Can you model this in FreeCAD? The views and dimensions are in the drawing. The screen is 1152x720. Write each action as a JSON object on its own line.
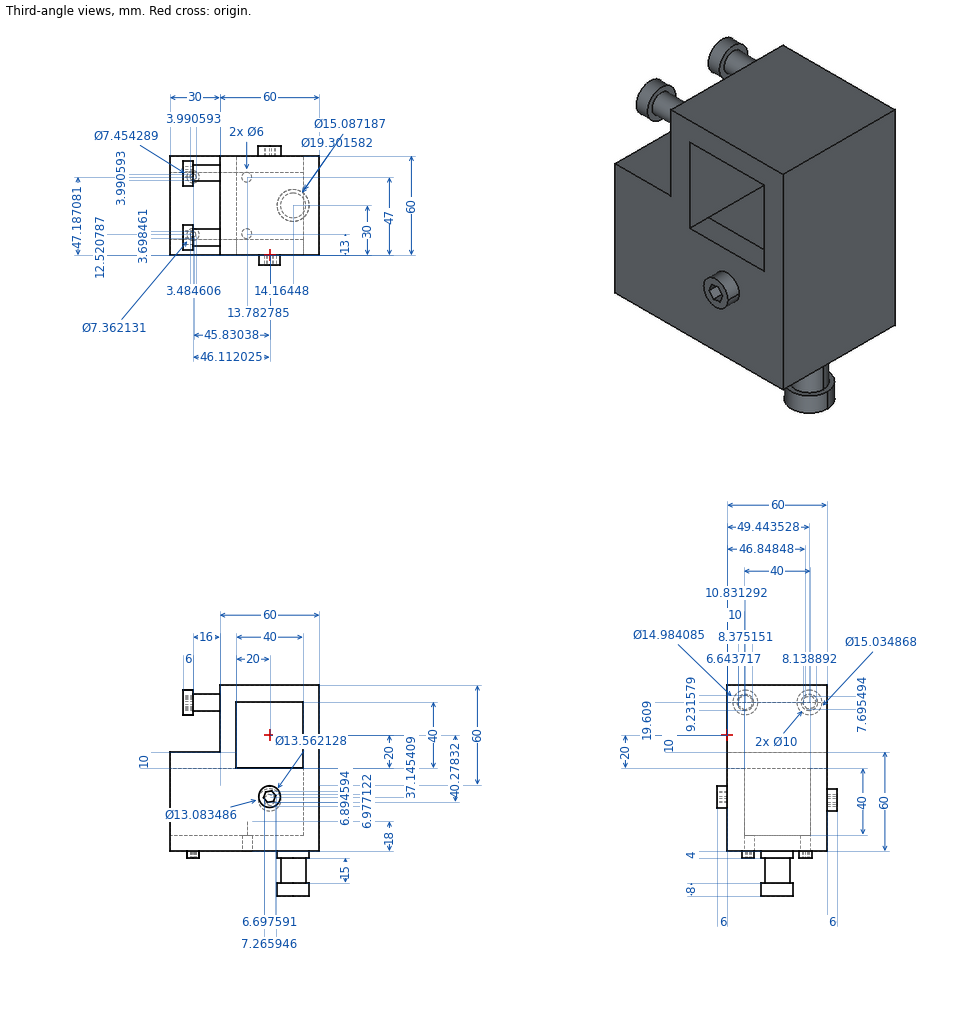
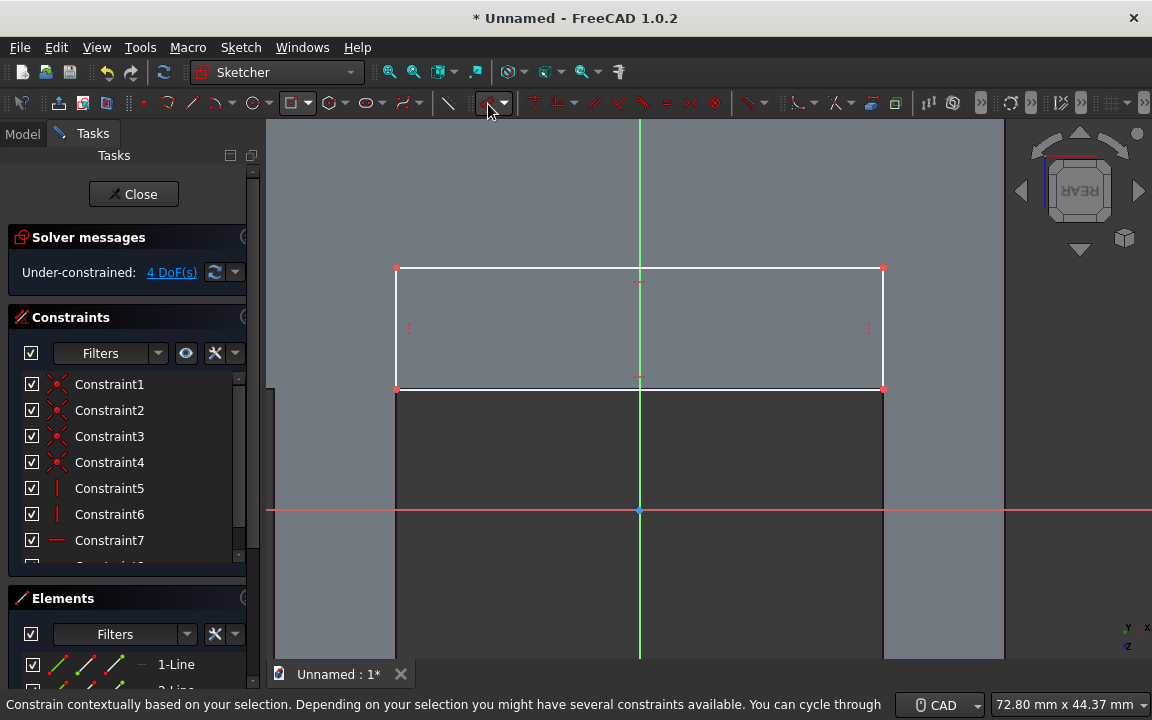
{"action": "left_click", "coordinate": [396, 305]}
{"action": "left_click", "coordinate": [362, 329]}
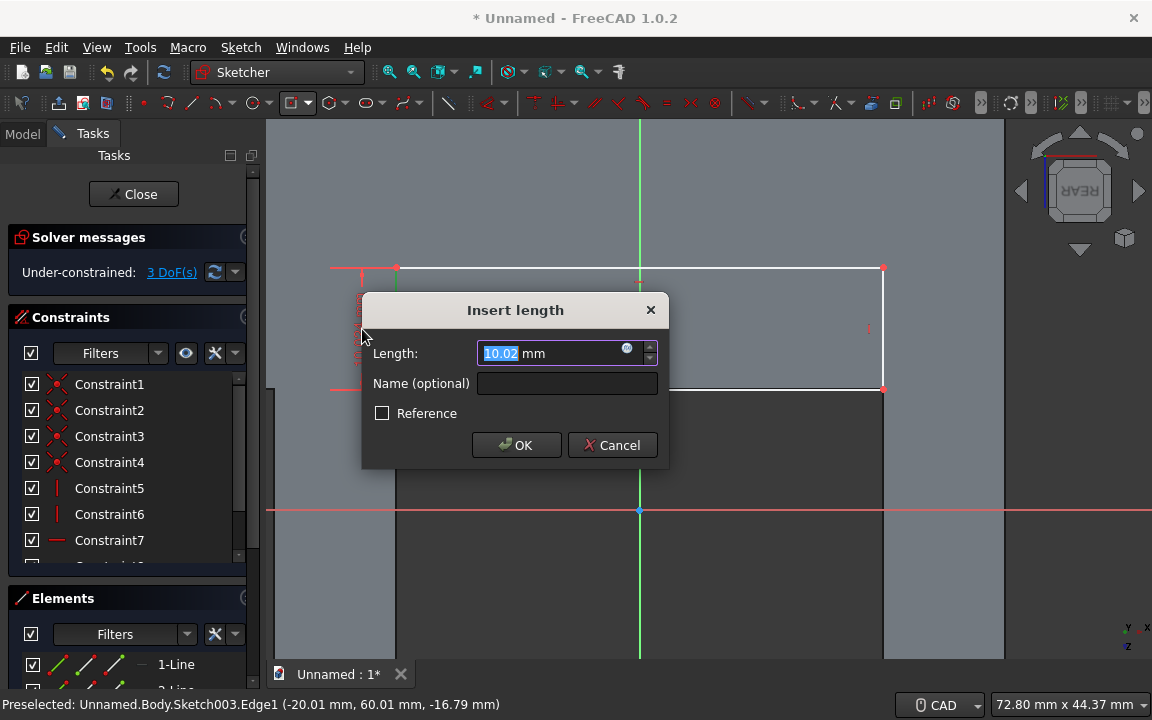
{"action": "type", "text": "10"}
{"action": "key", "text": "Return"}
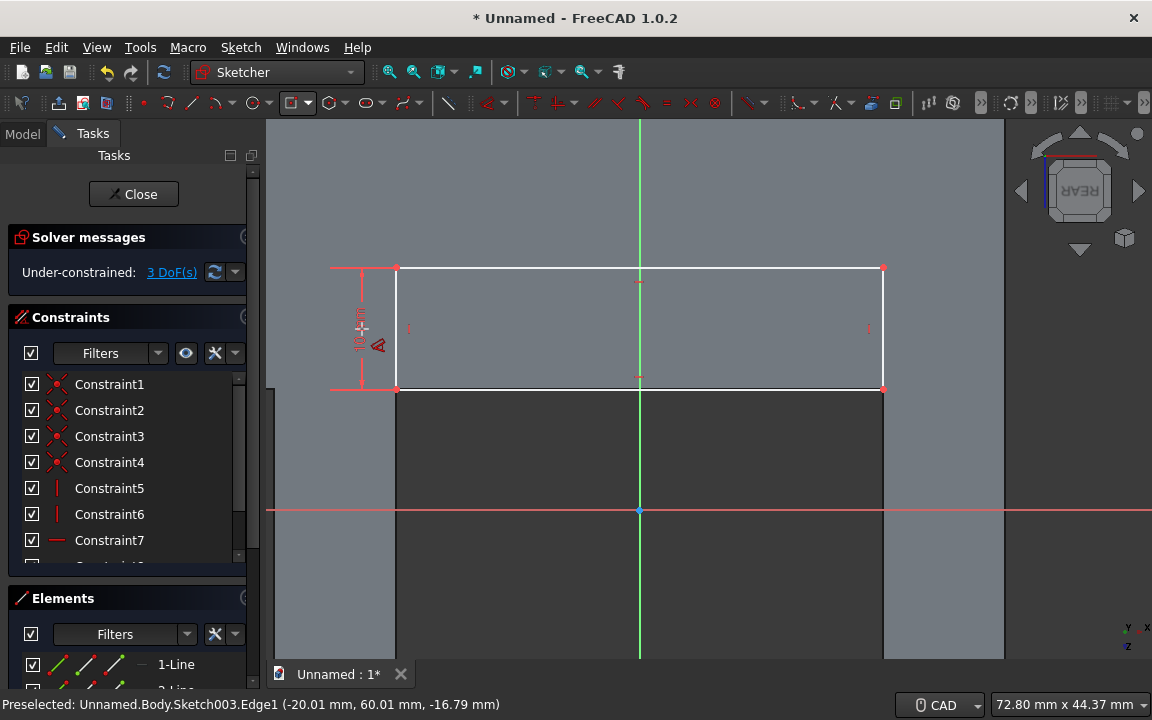
{"action": "left_click", "coordinate": [542, 390]}
{"action": "left_click", "coordinate": [527, 424]}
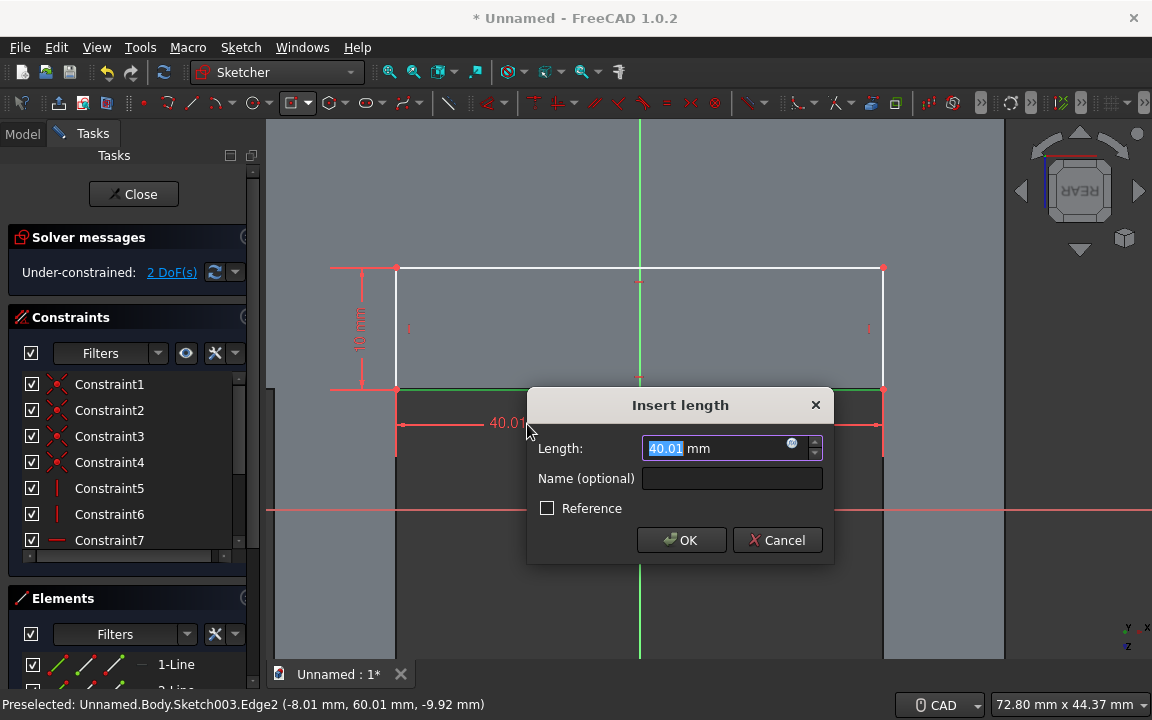
{"action": "type", "text": "40"}
{"action": "key", "text": "Return"}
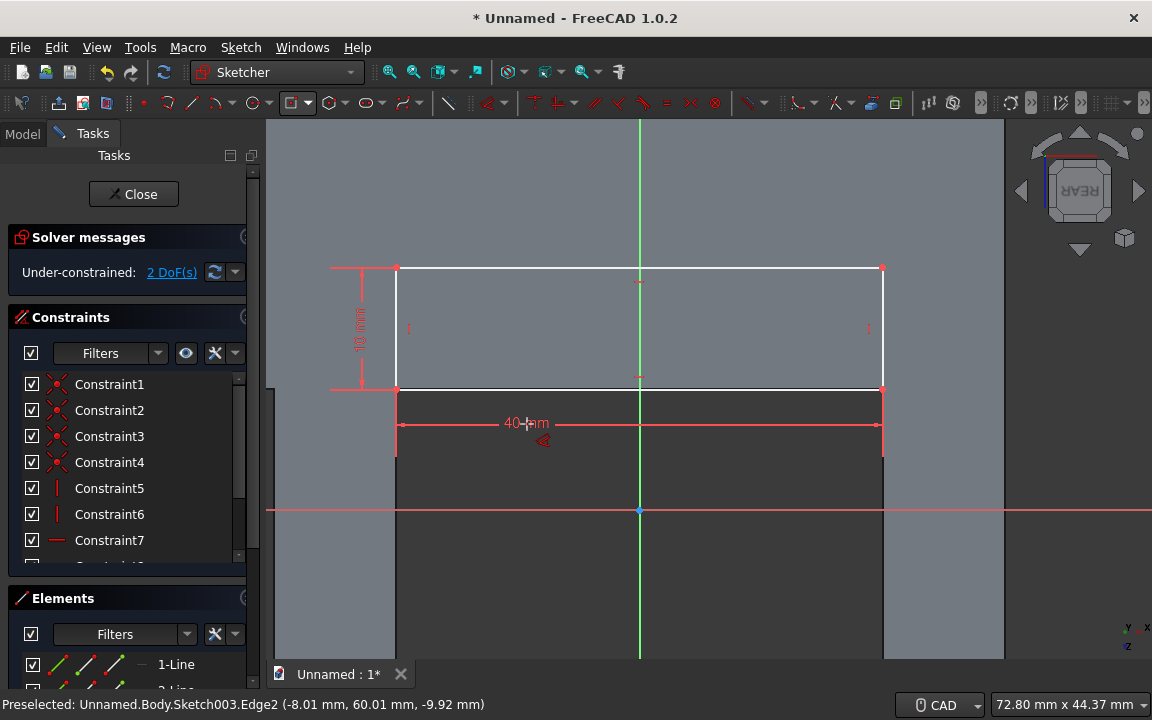
{"action": "left_click", "coordinate": [396, 268]}
{"action": "left_click", "coordinate": [518, 544]}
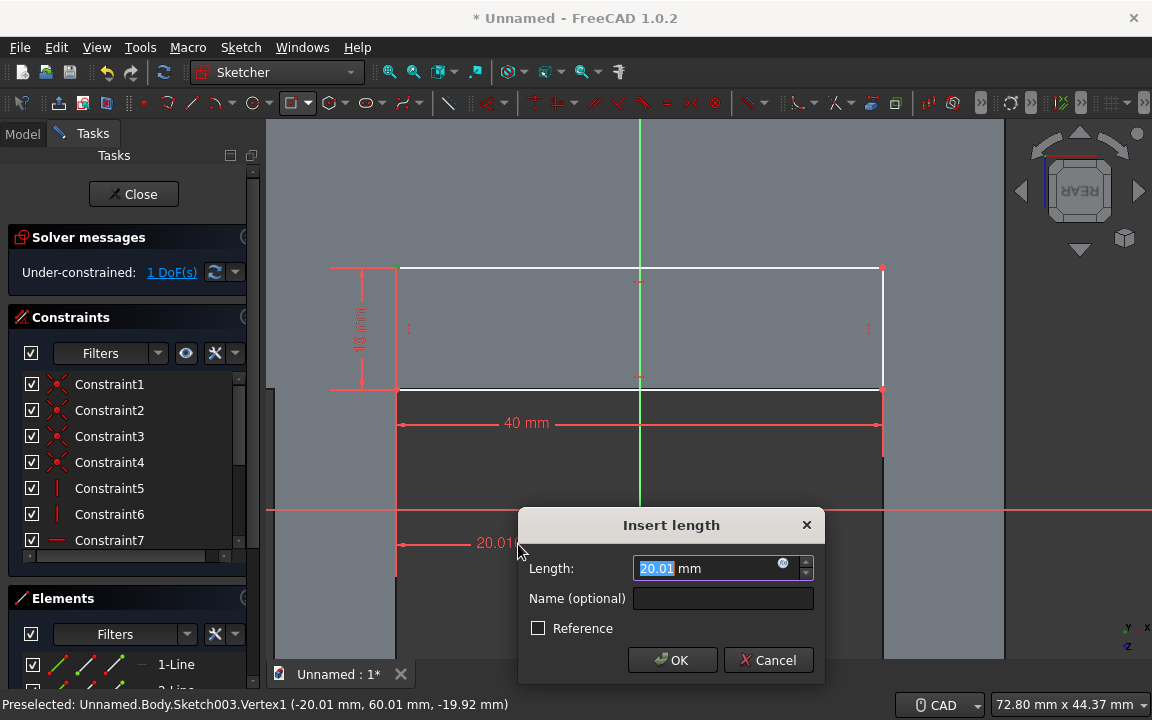
{"action": "type", "text": "20"}
{"action": "key", "text": "Return"}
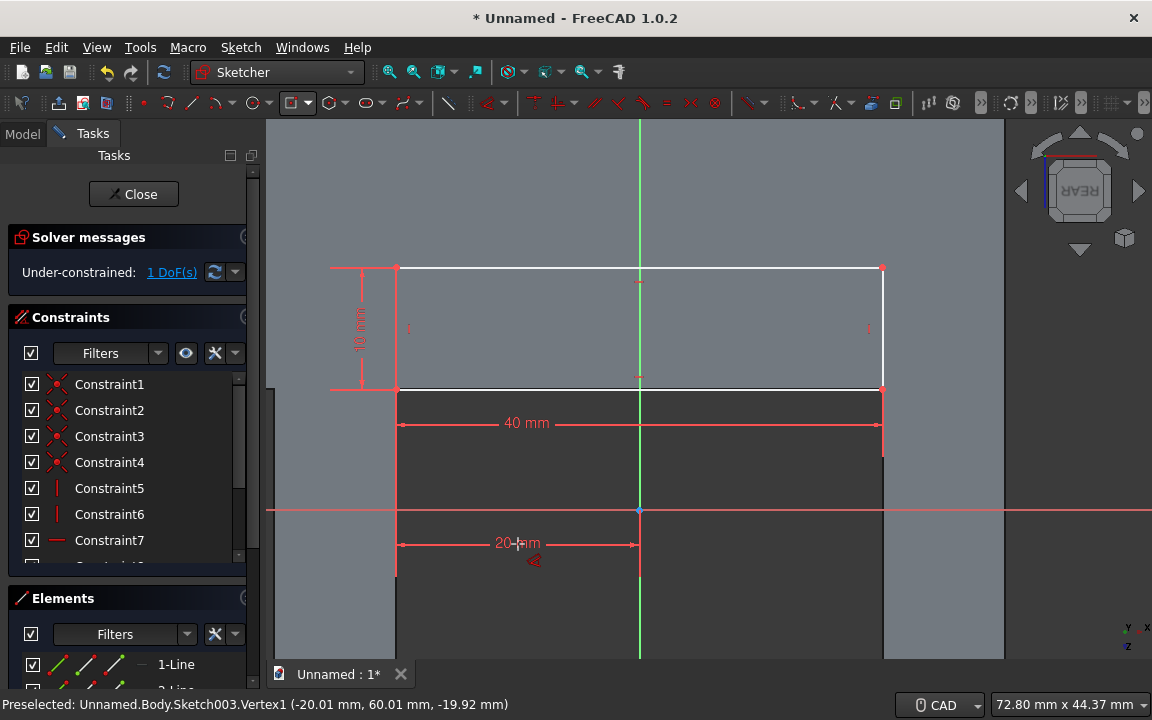
{"action": "left_click", "coordinate": [396, 268]}
{"action": "left_click", "coordinate": [362, 389]}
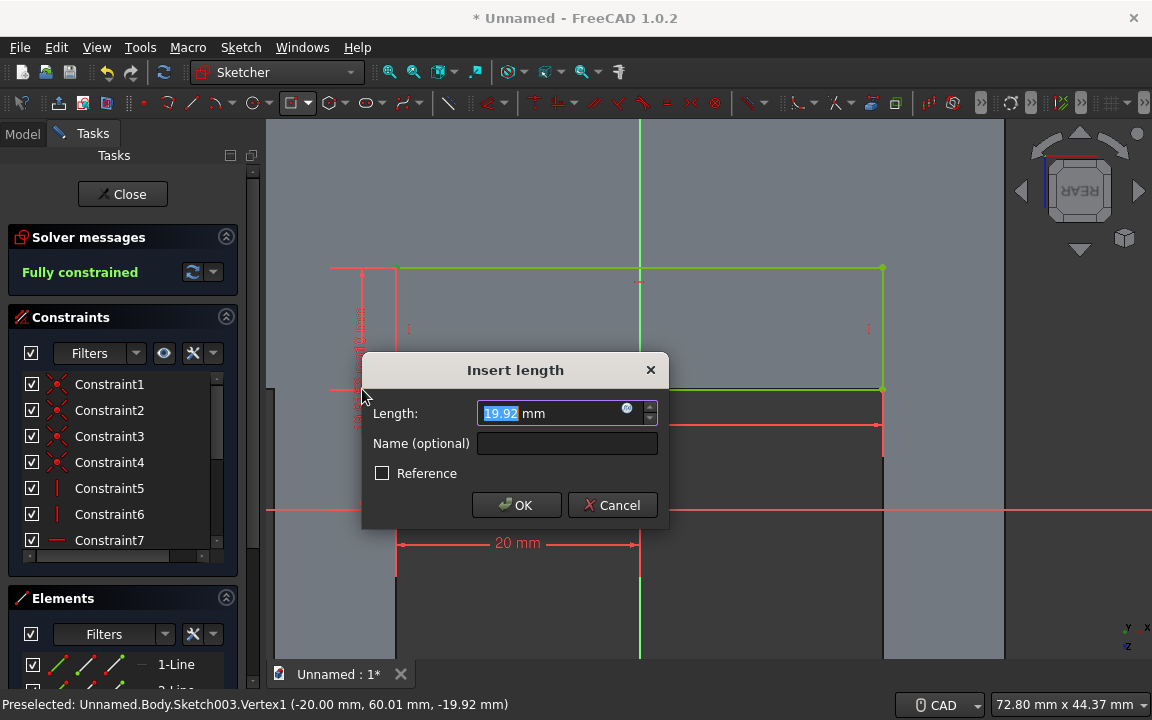
{"action": "type", "text": "20"}
{"action": "key", "text": "Return"}
{"action": "key", "text": "Escape"}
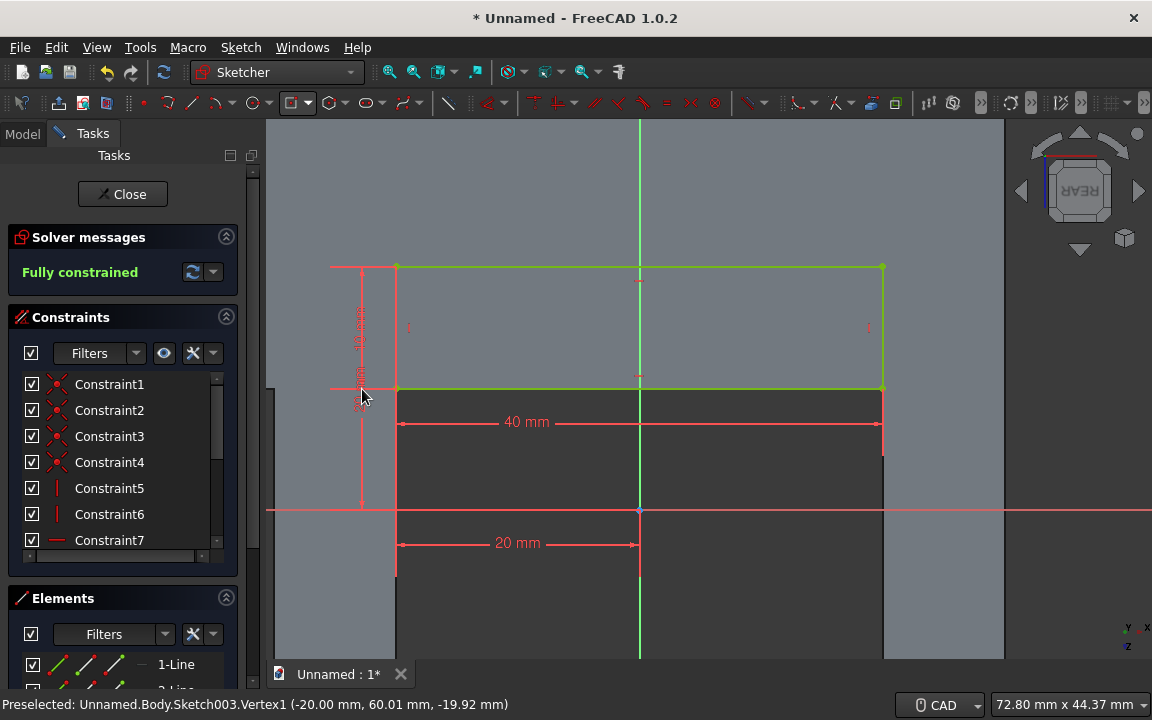
{"action": "left_click", "coordinate": [123, 194]}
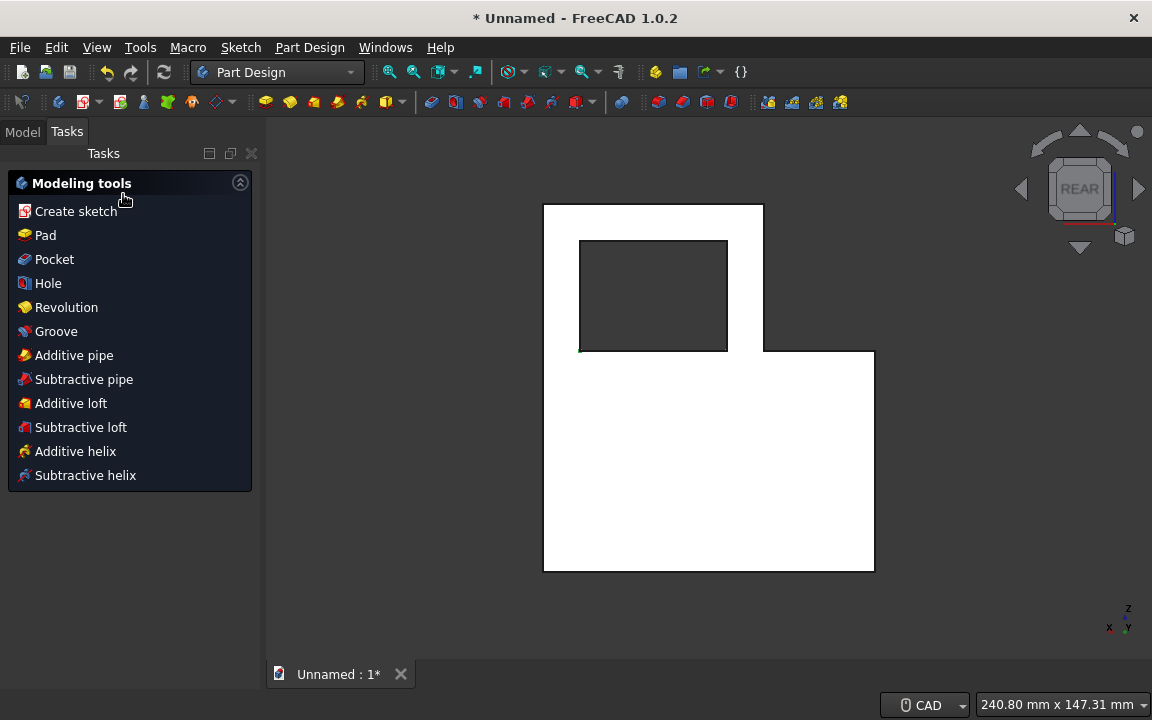
{"action": "left_click", "coordinate": [432, 102]}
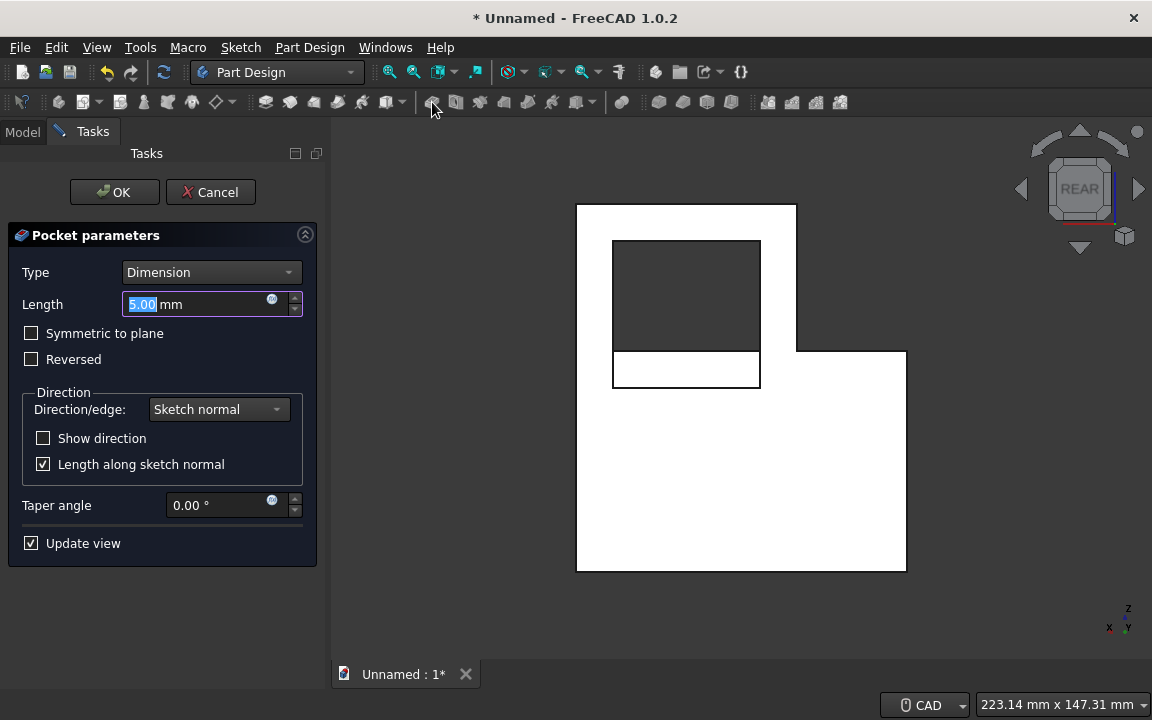
{"action": "type", "text": "60"}
{"action": "key", "text": "Tab"}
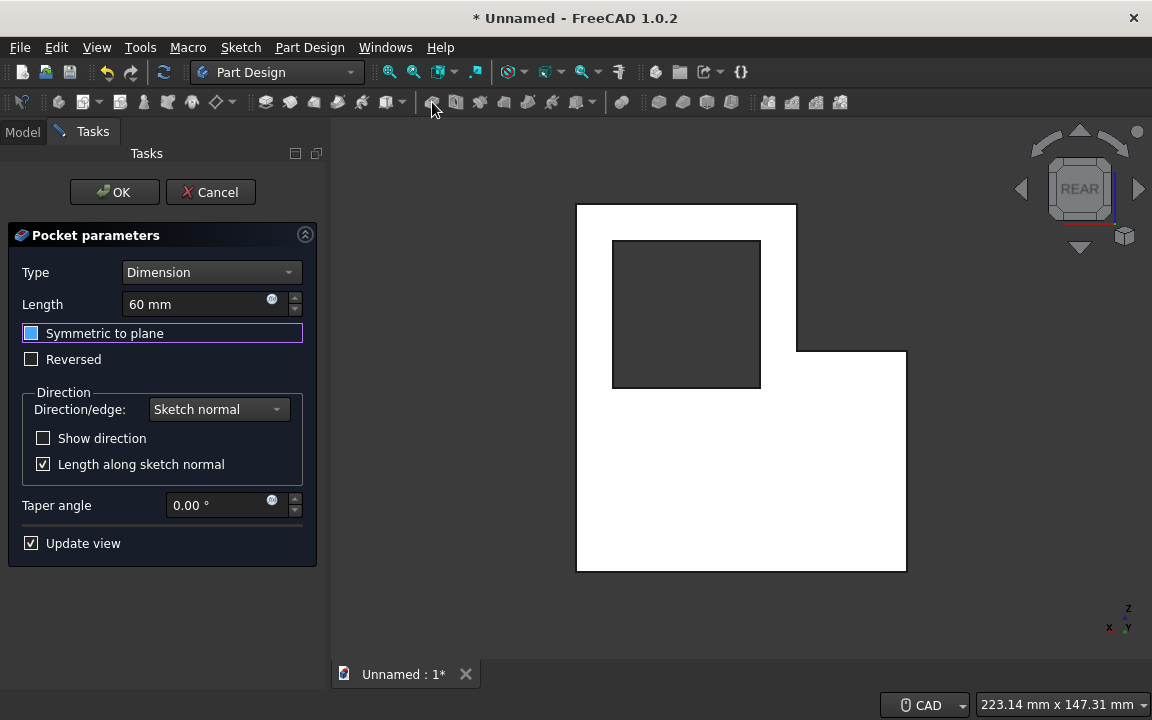
{"action": "left_click", "coordinate": [115, 192]}